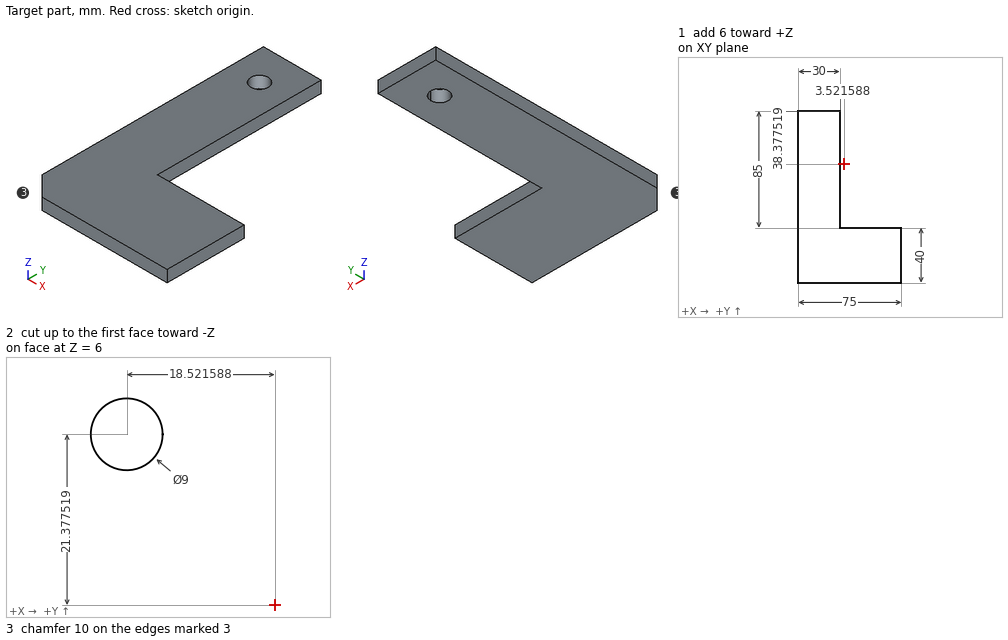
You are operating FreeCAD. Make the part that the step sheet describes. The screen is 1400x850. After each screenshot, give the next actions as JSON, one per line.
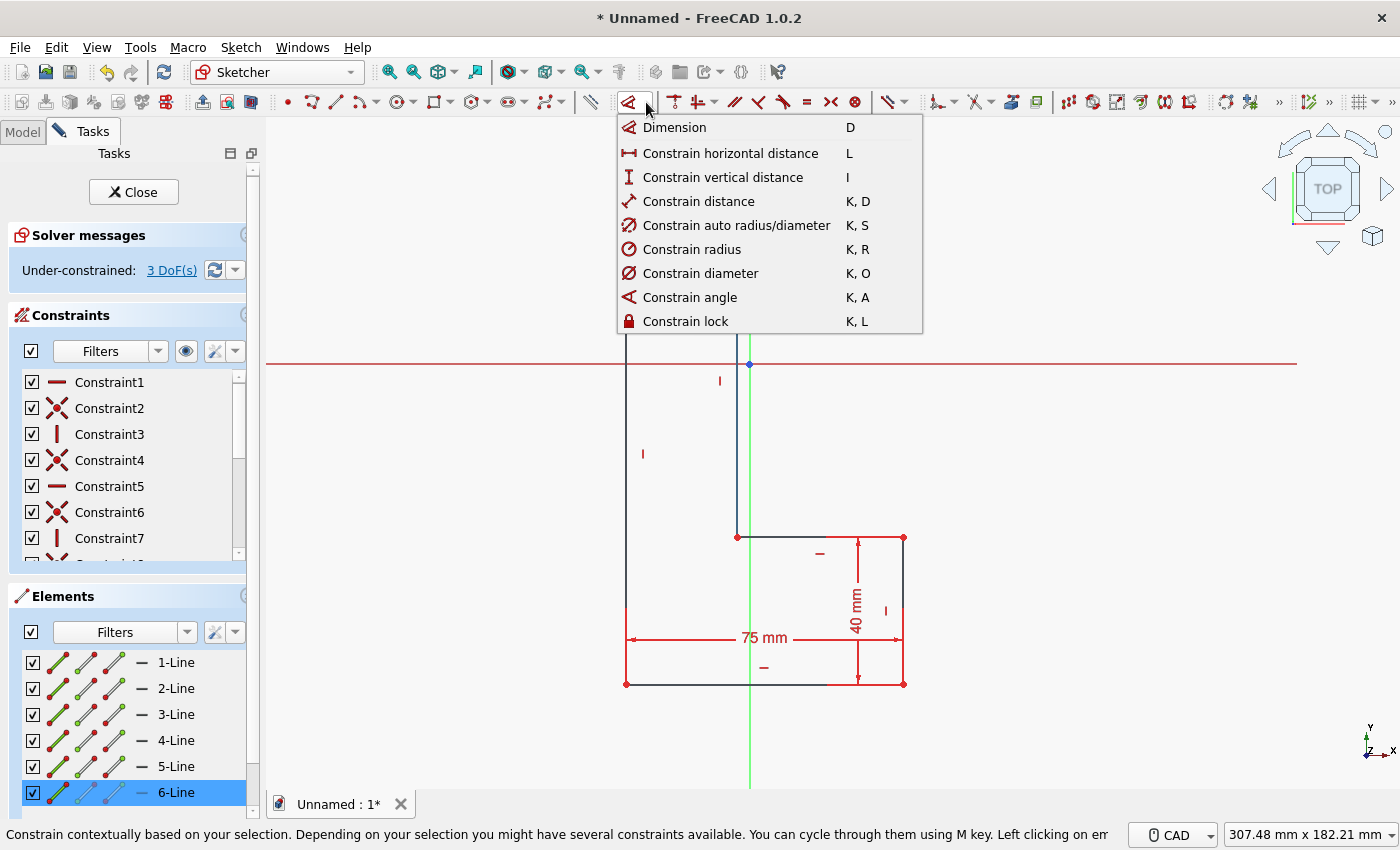
{"action": "left_click", "coordinate": [770, 177]}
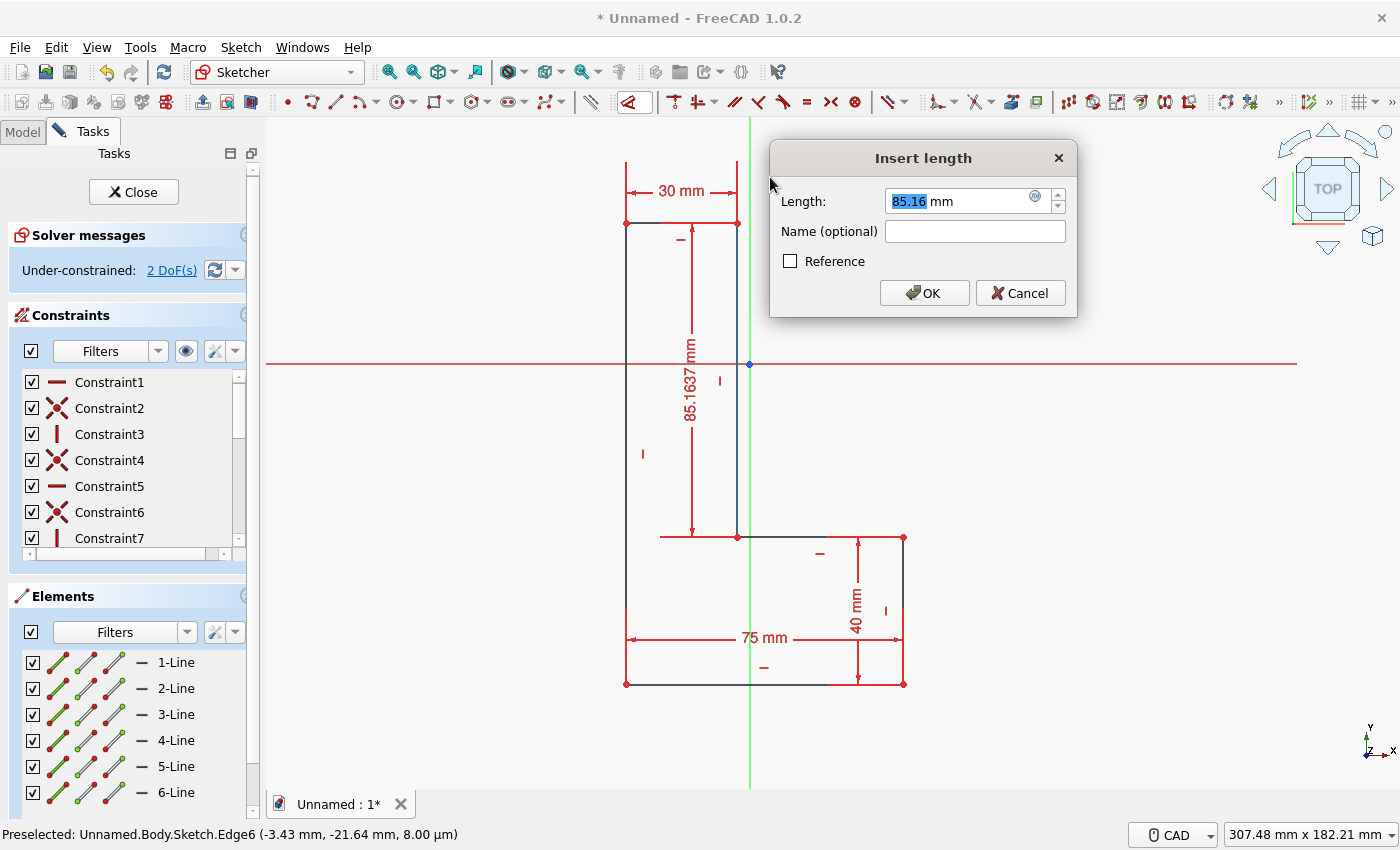
{"action": "type", "text": "85"}
{"action": "key", "text": "Return"}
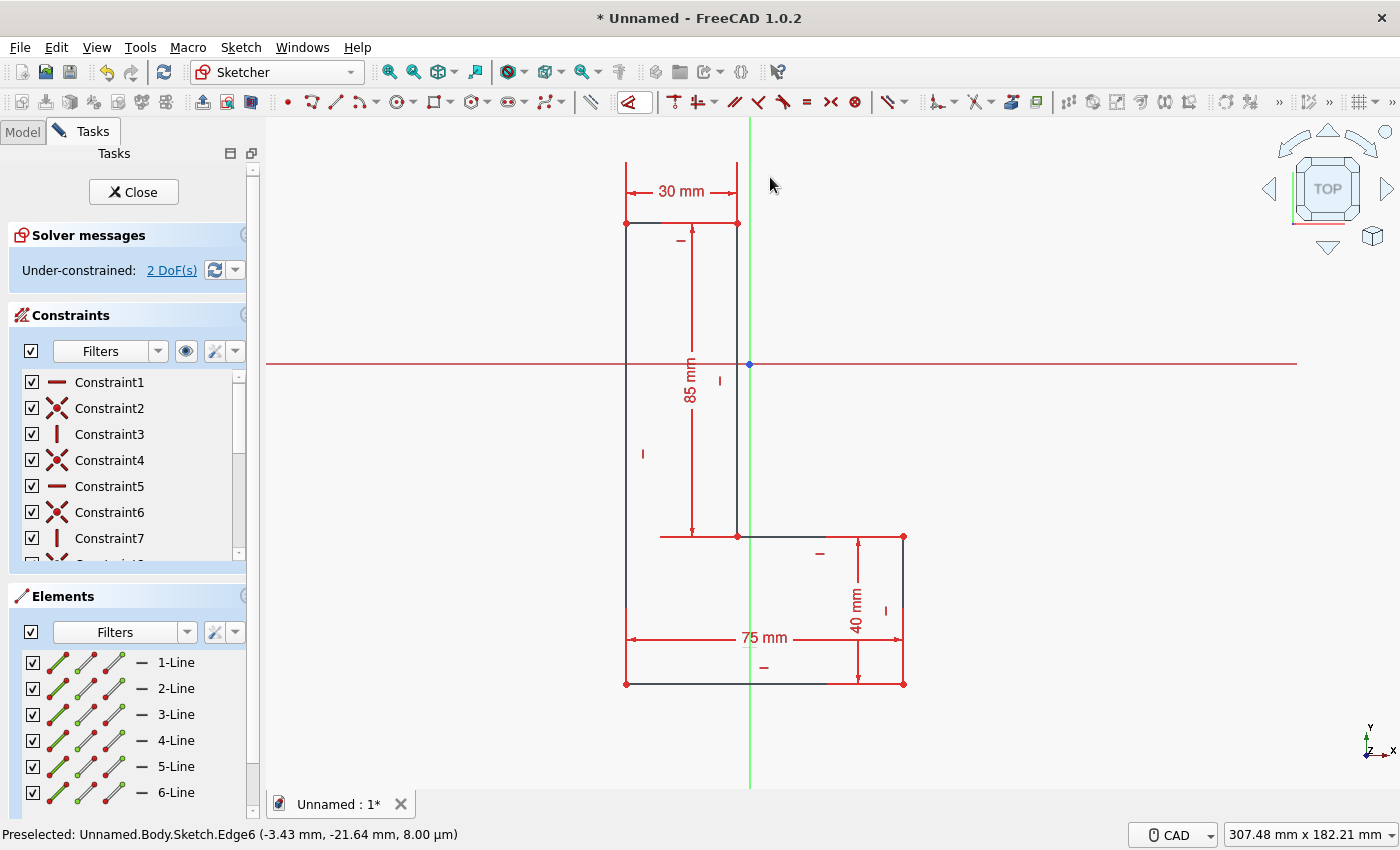
{"action": "scroll", "coordinate": [737, 223], "scroll_direction": "up", "scroll_amount": 6}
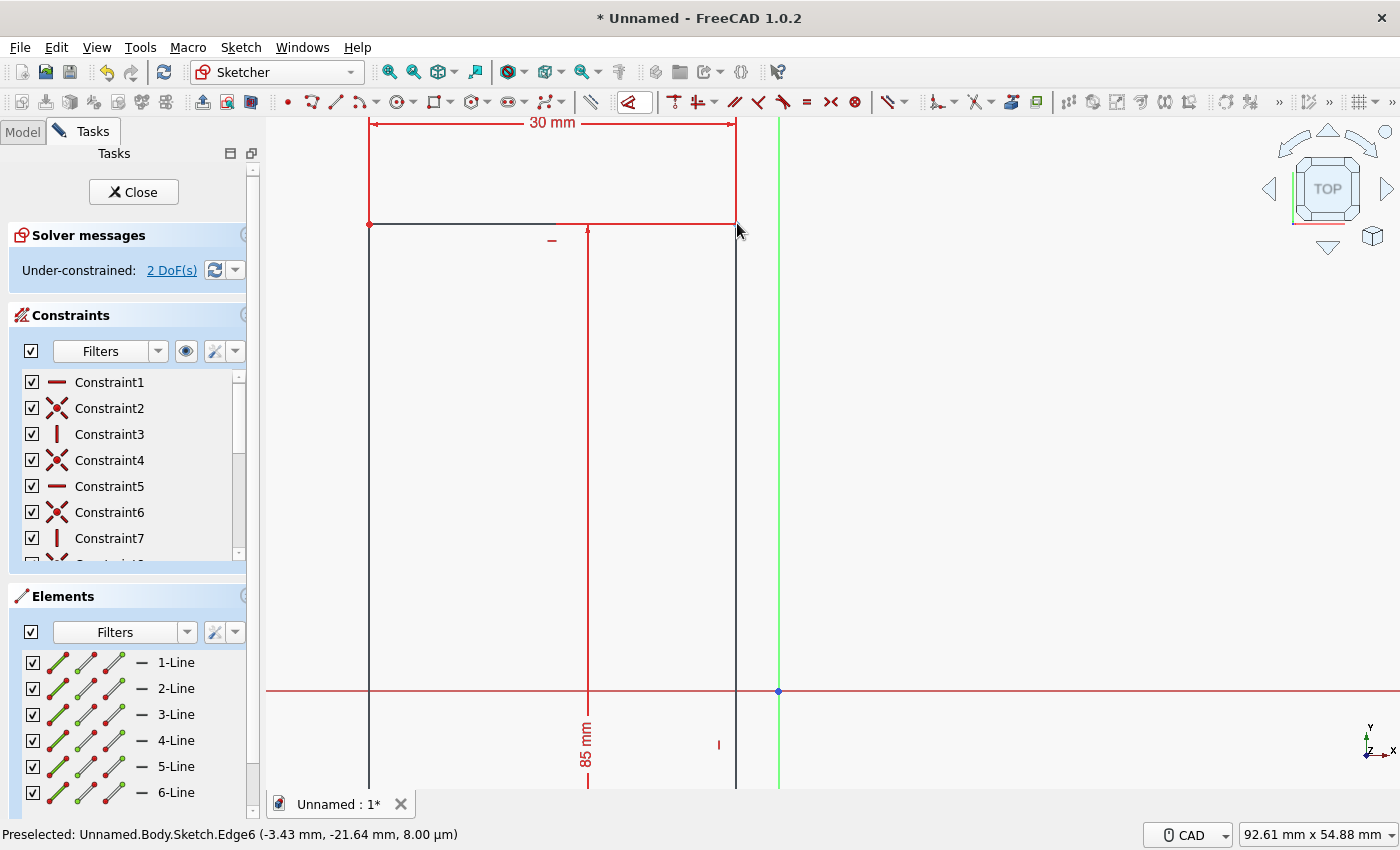
{"action": "left_click", "coordinate": [736, 224]}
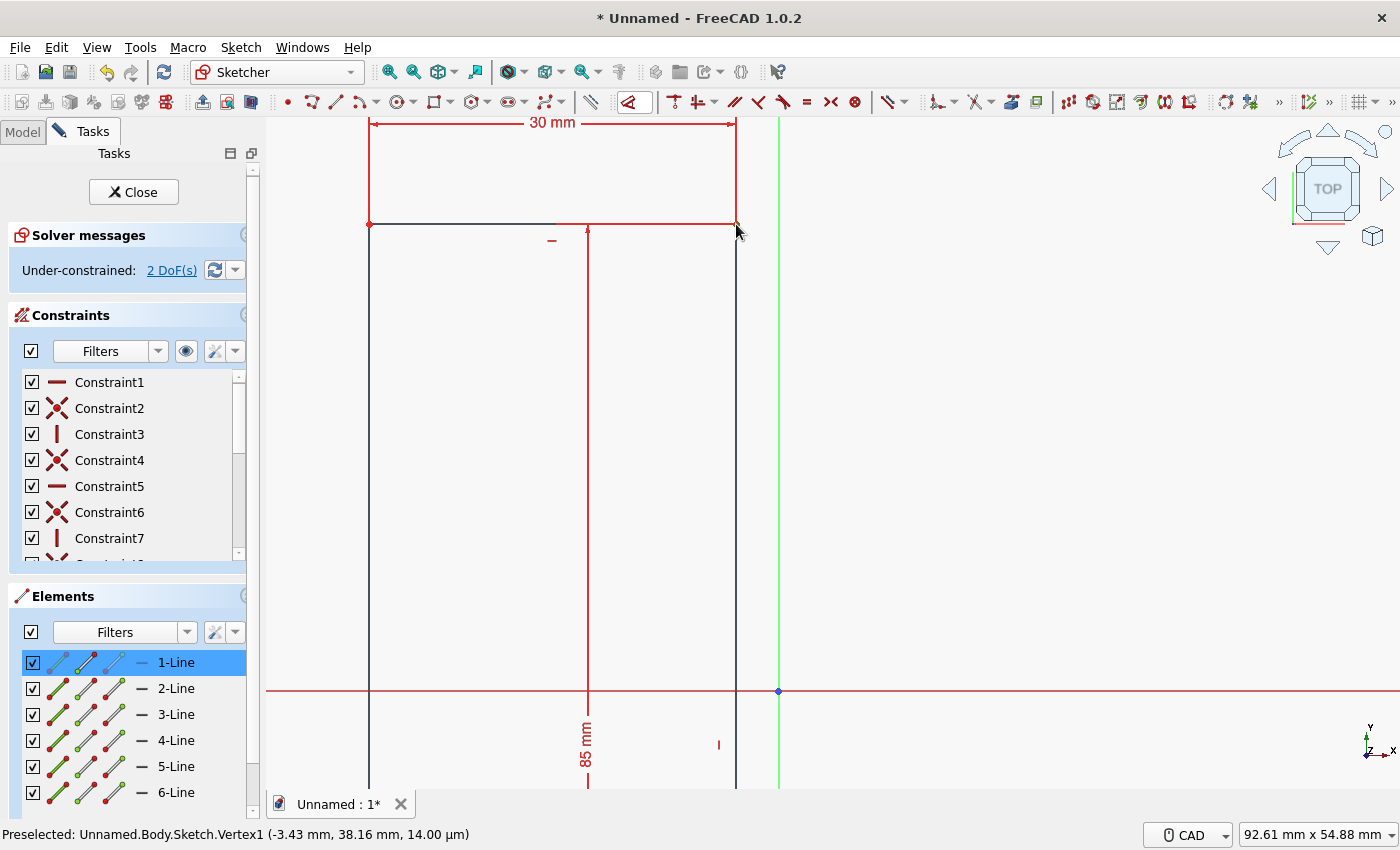
{"action": "key", "text": "l"}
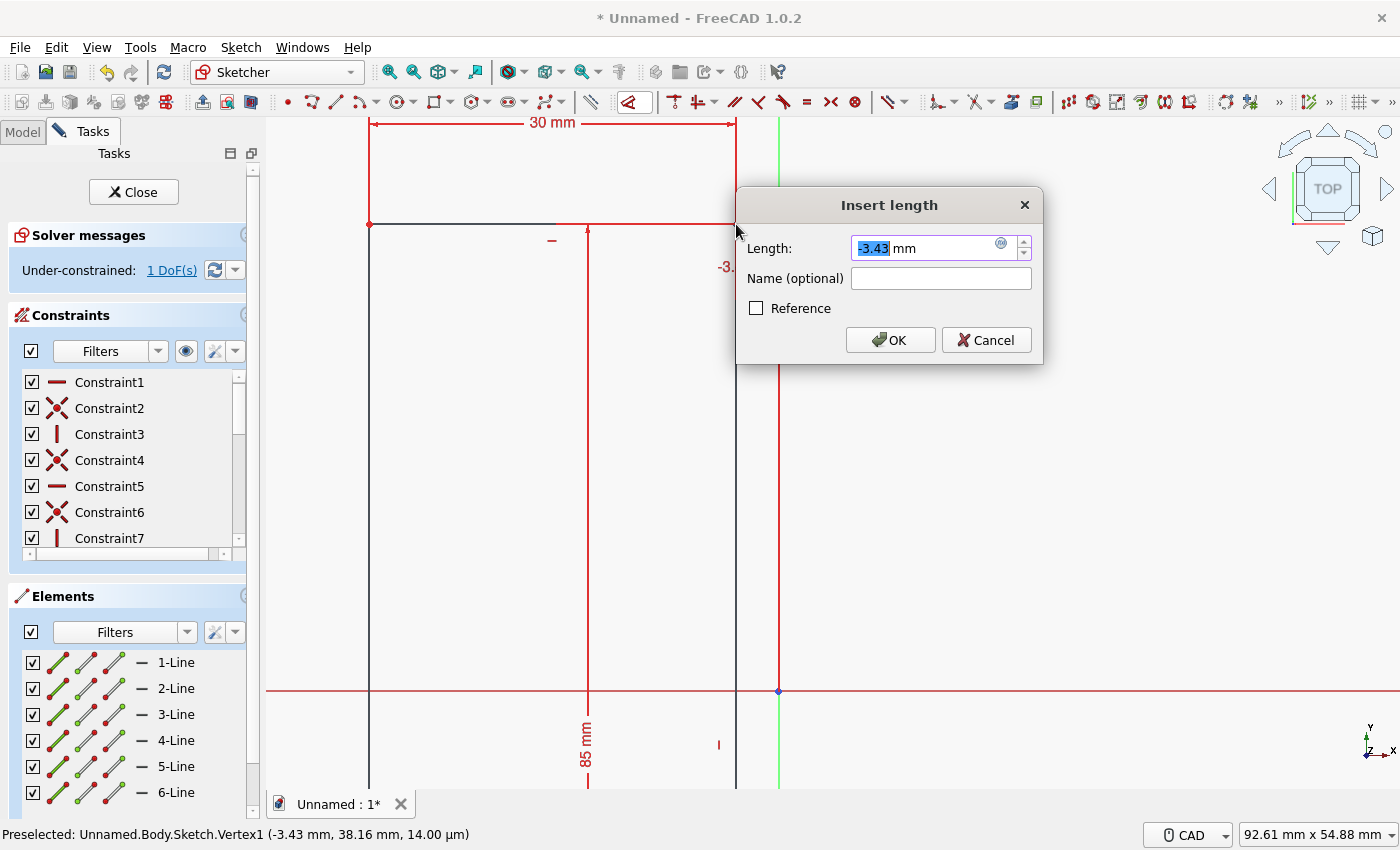
{"action": "type", "text": "-3.521588"}
{"action": "key", "text": "Return"}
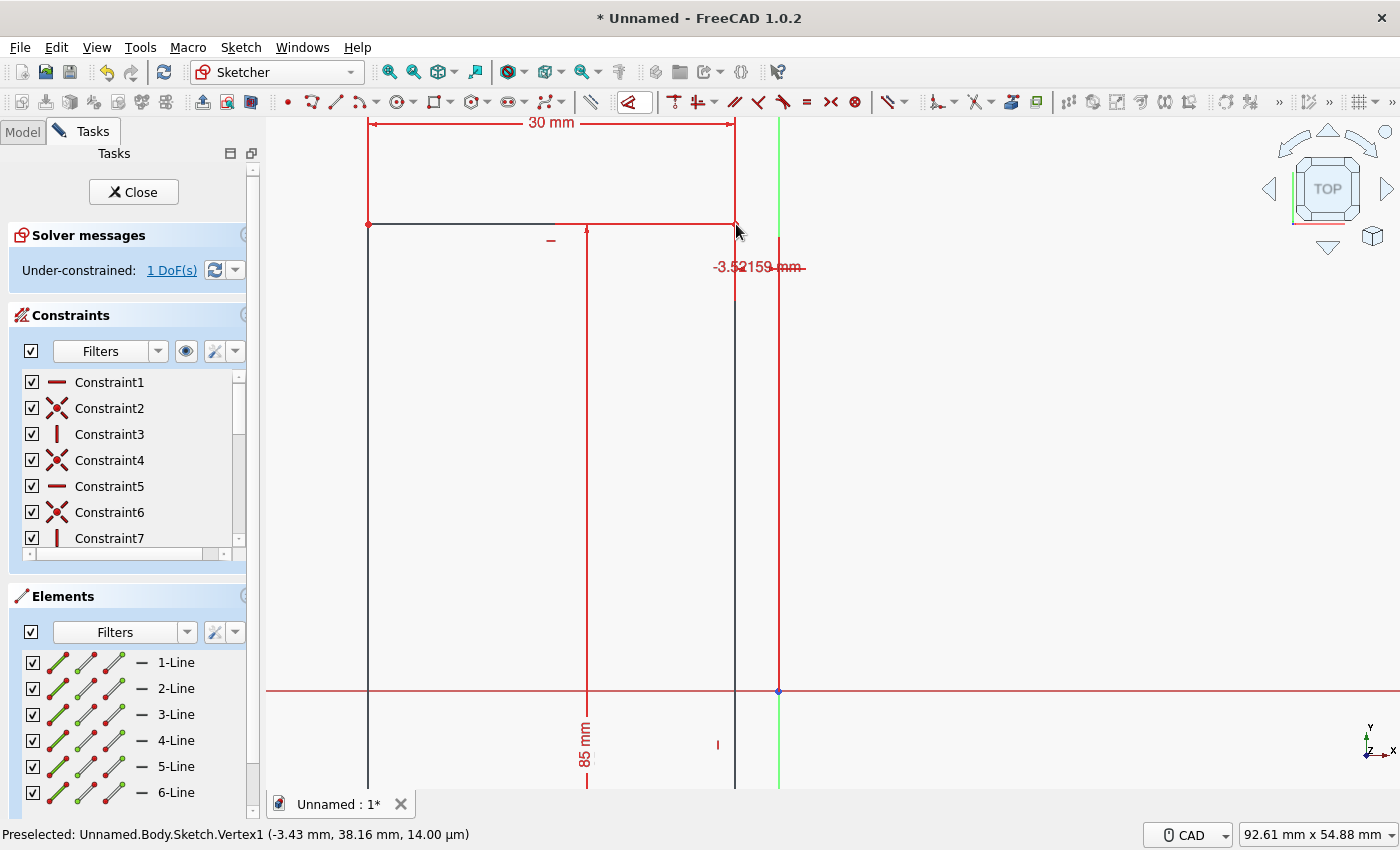
{"action": "left_click", "coordinate": [735, 224]}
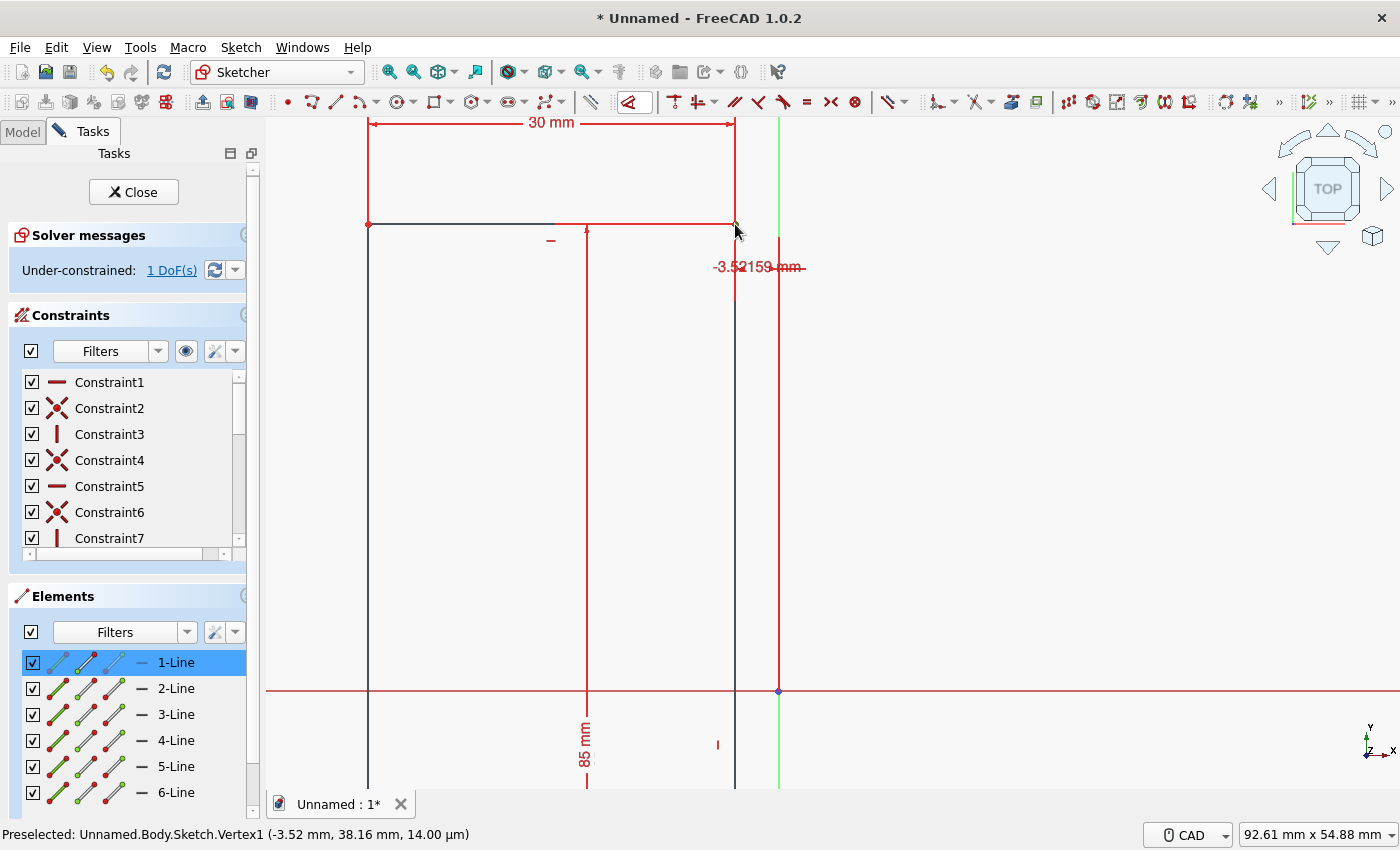
{"action": "left_click", "coordinate": [646, 102]}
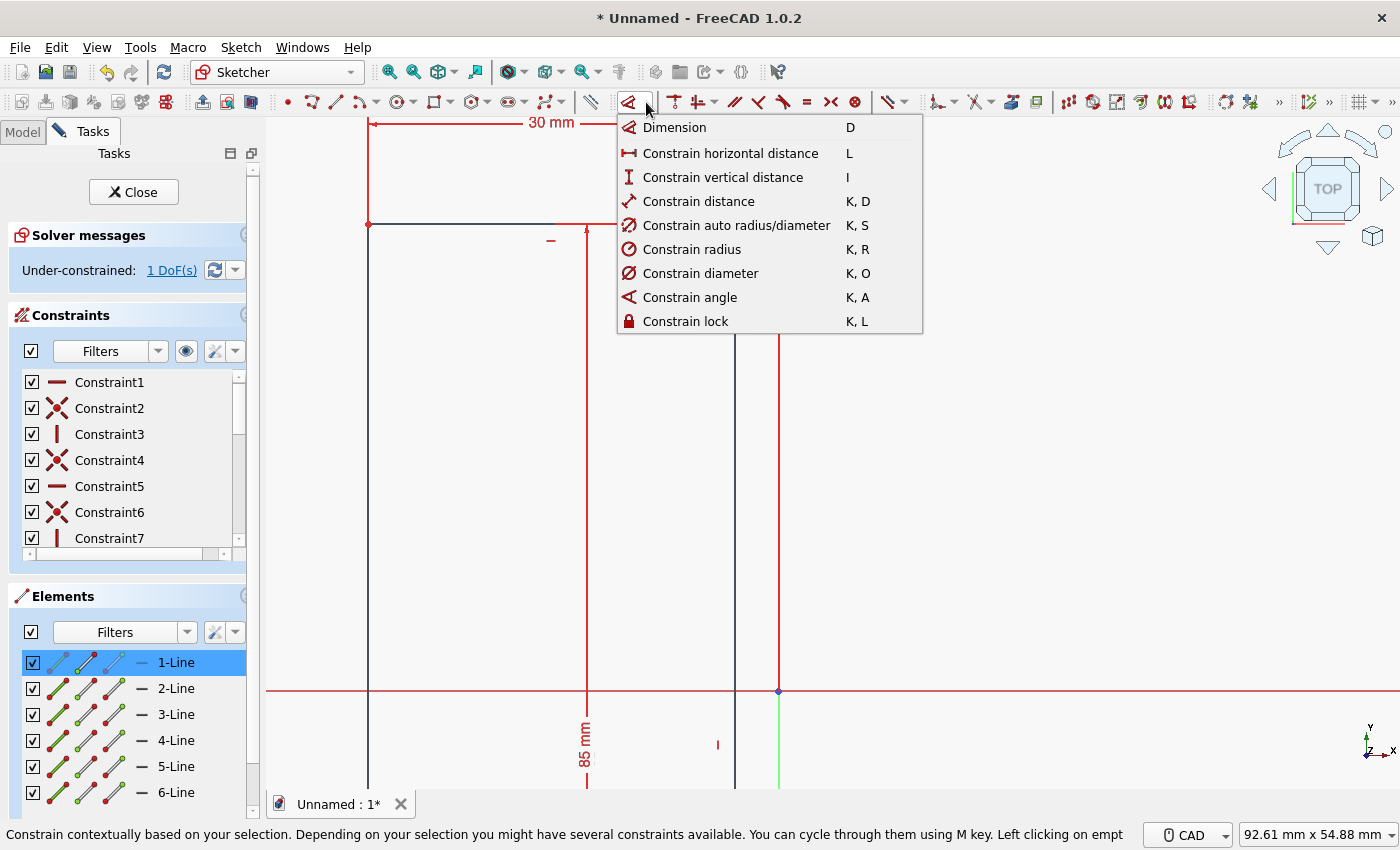
{"action": "left_click", "coordinate": [770, 177]}